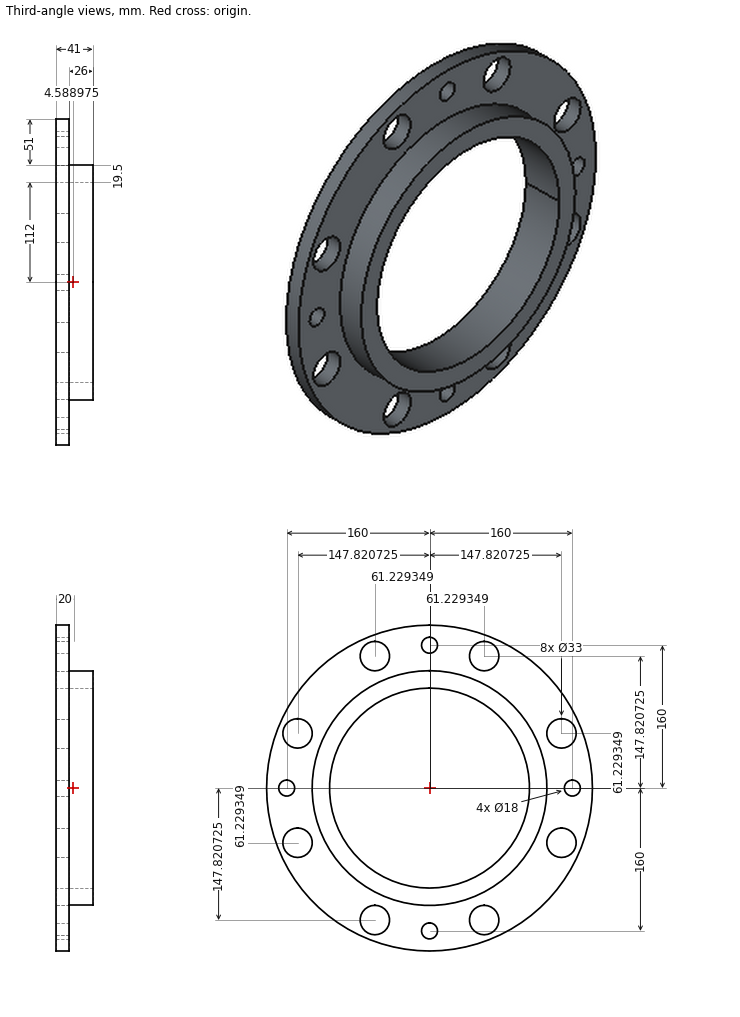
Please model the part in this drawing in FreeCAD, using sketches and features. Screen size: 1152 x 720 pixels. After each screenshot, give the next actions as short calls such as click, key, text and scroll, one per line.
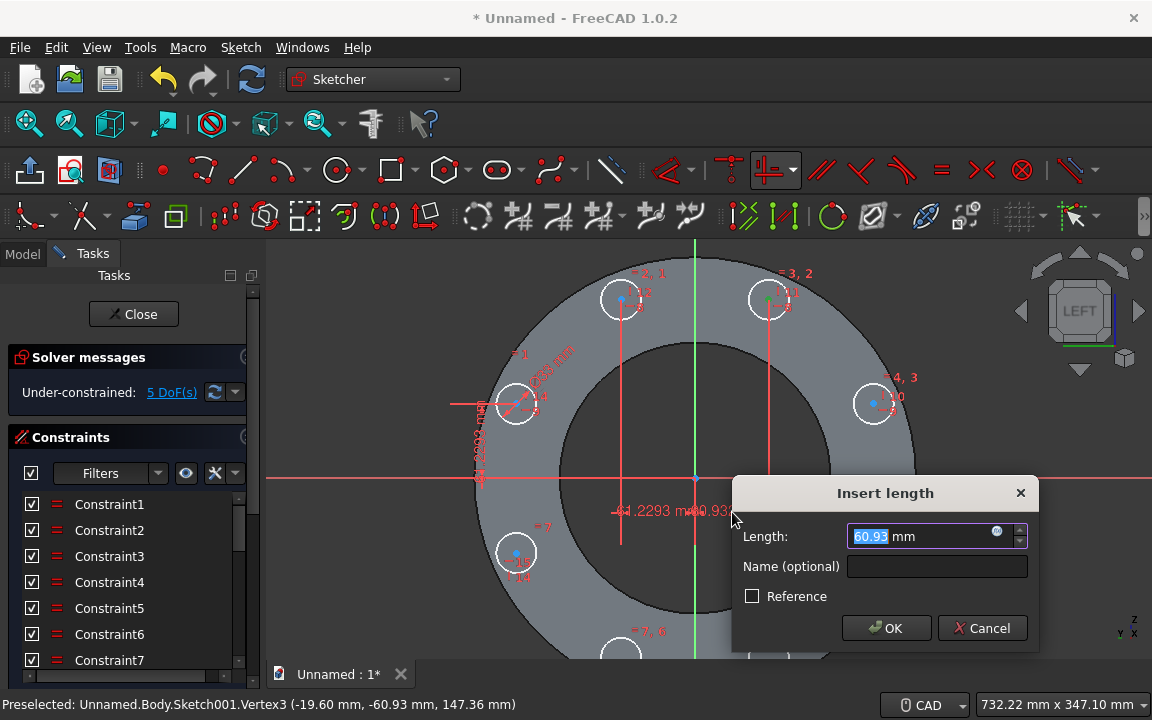
text(61.229349)
key(Return)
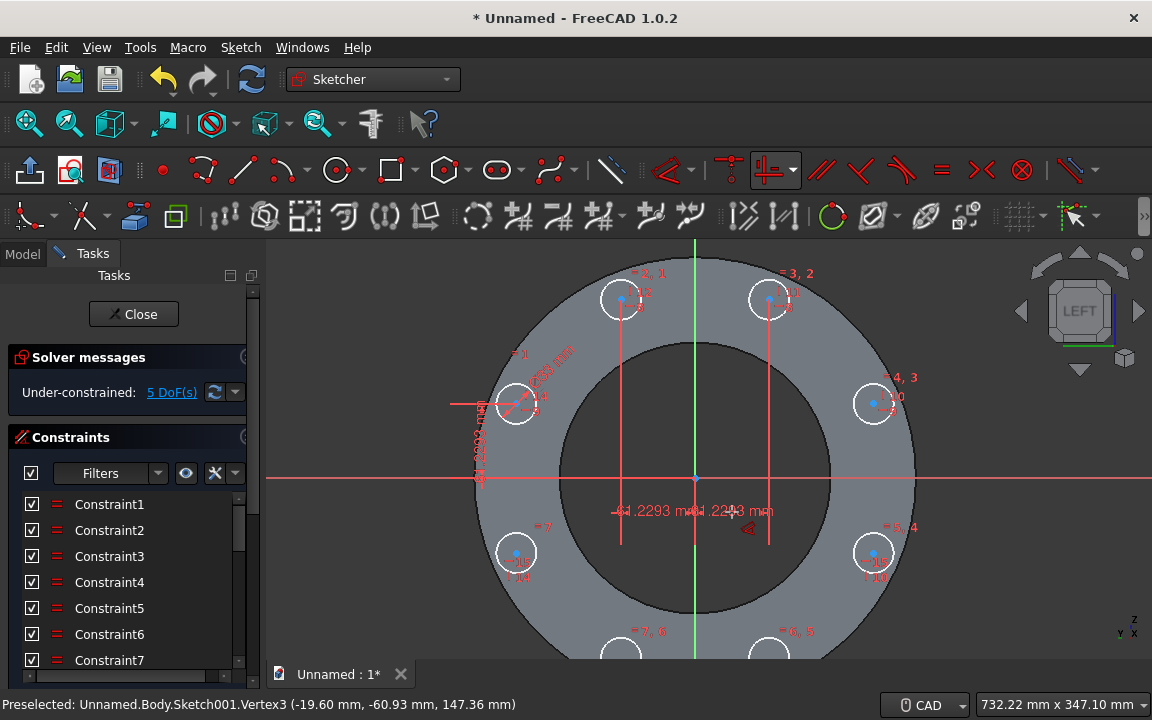
click(874, 553)
click(908, 516)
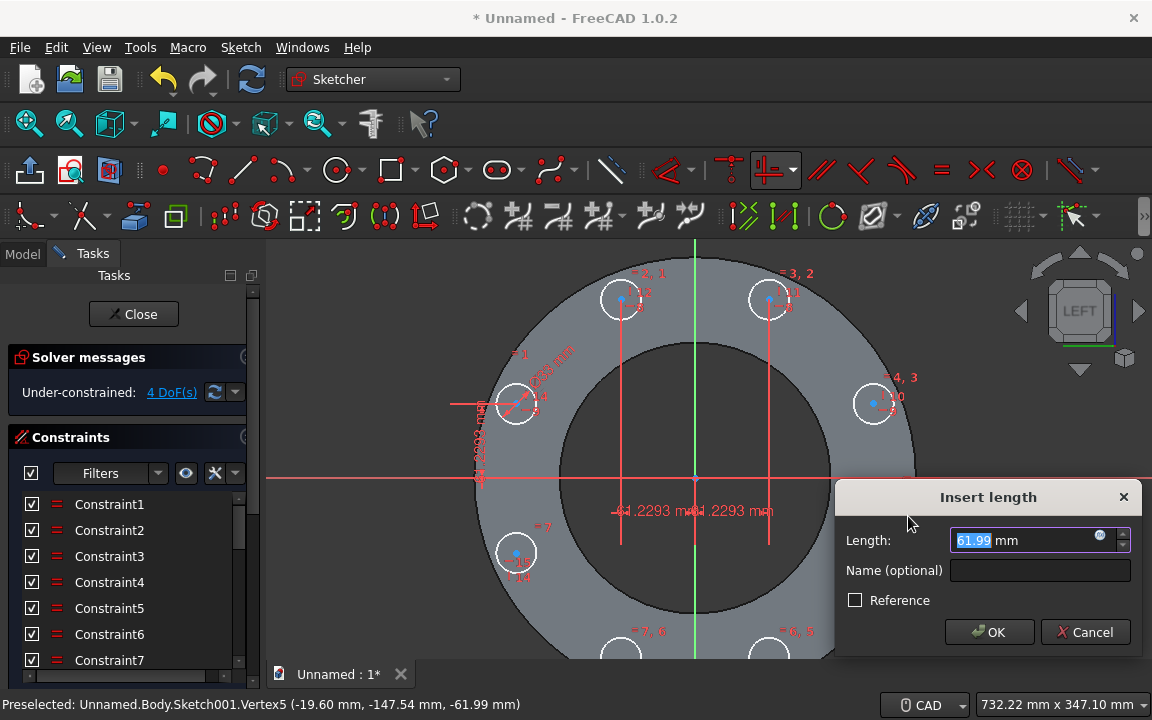
text(61.229349)
key(Return)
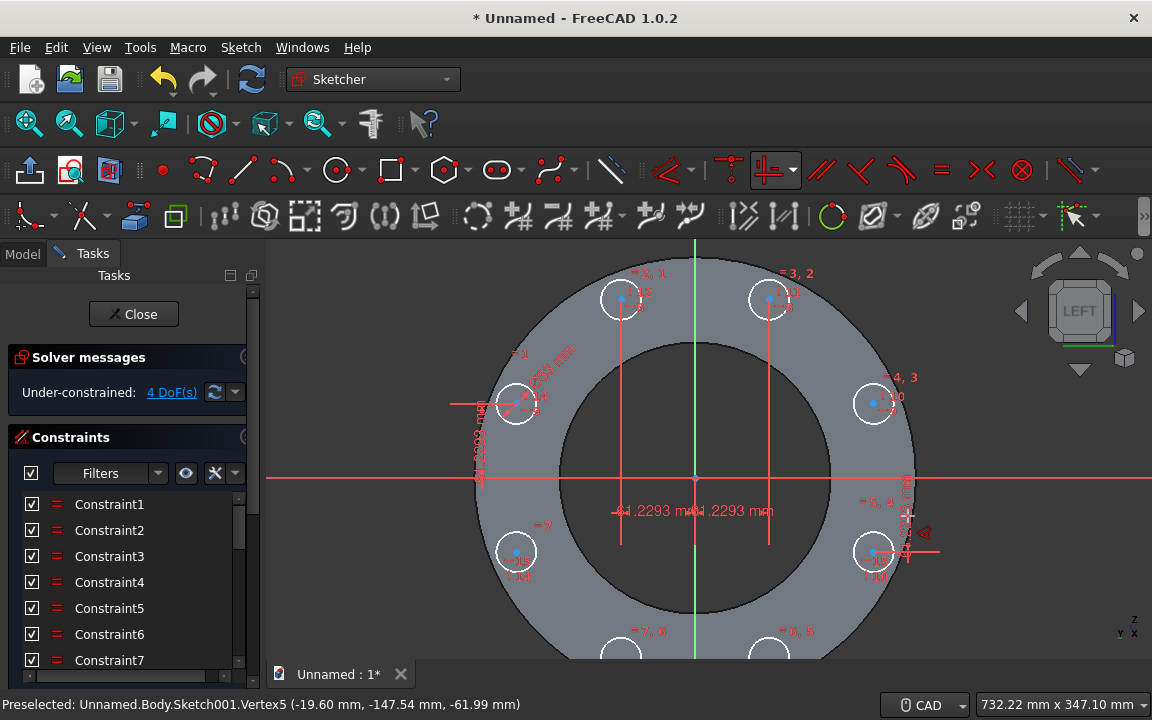
click(516, 404)
click(647, 370)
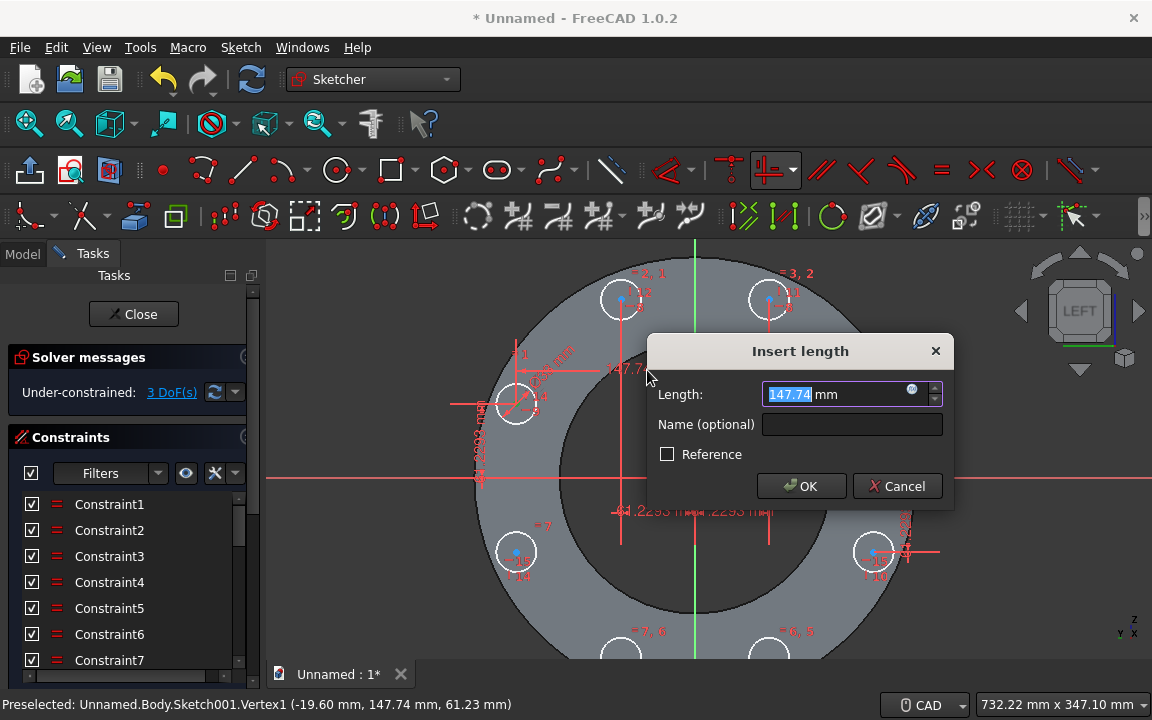
text(147.820725)
key(Return)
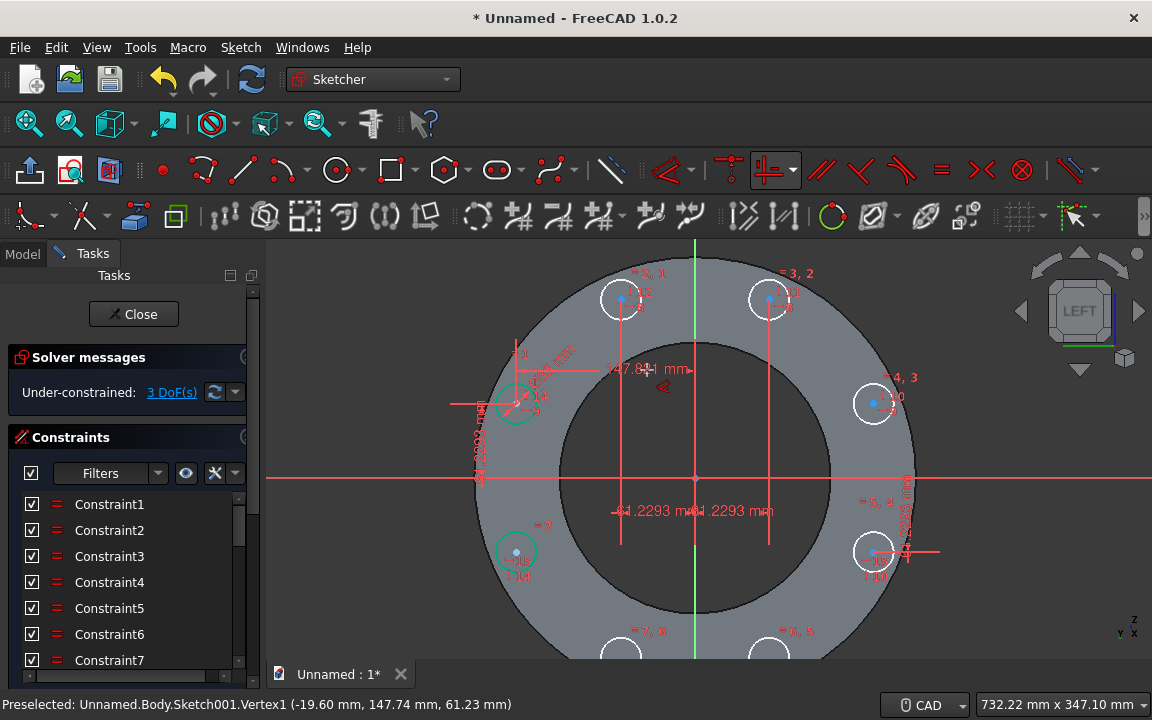
click(621, 300)
click(587, 348)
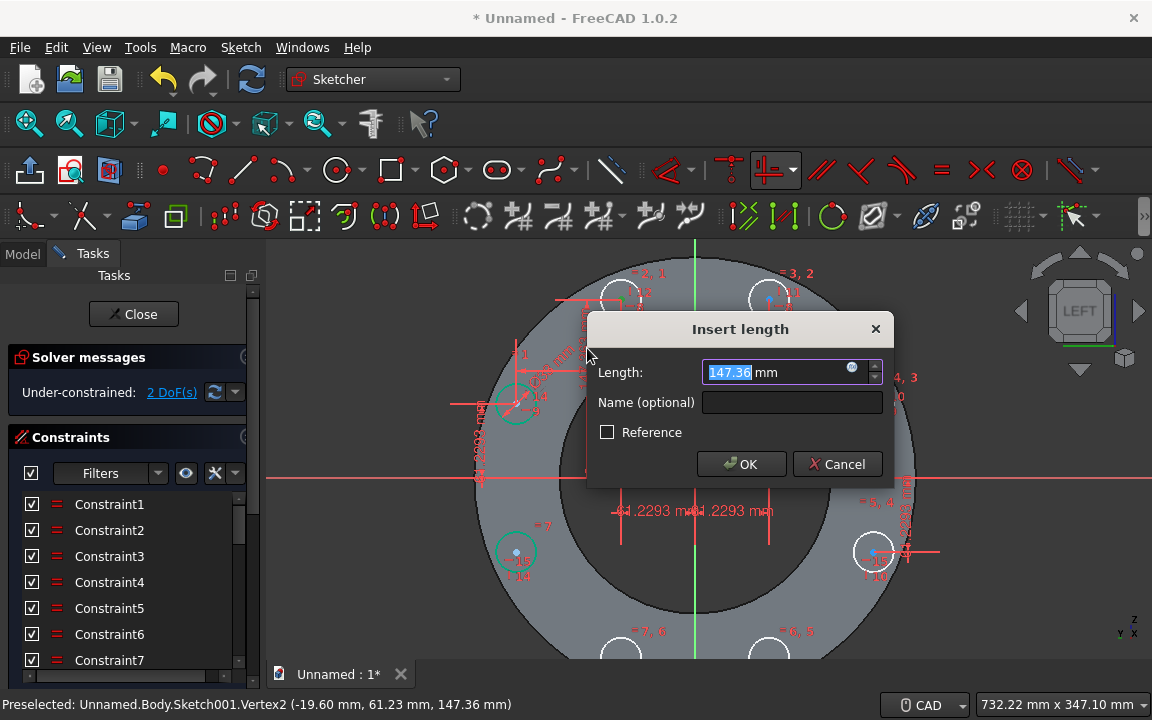
text(147.820725)
key(Return)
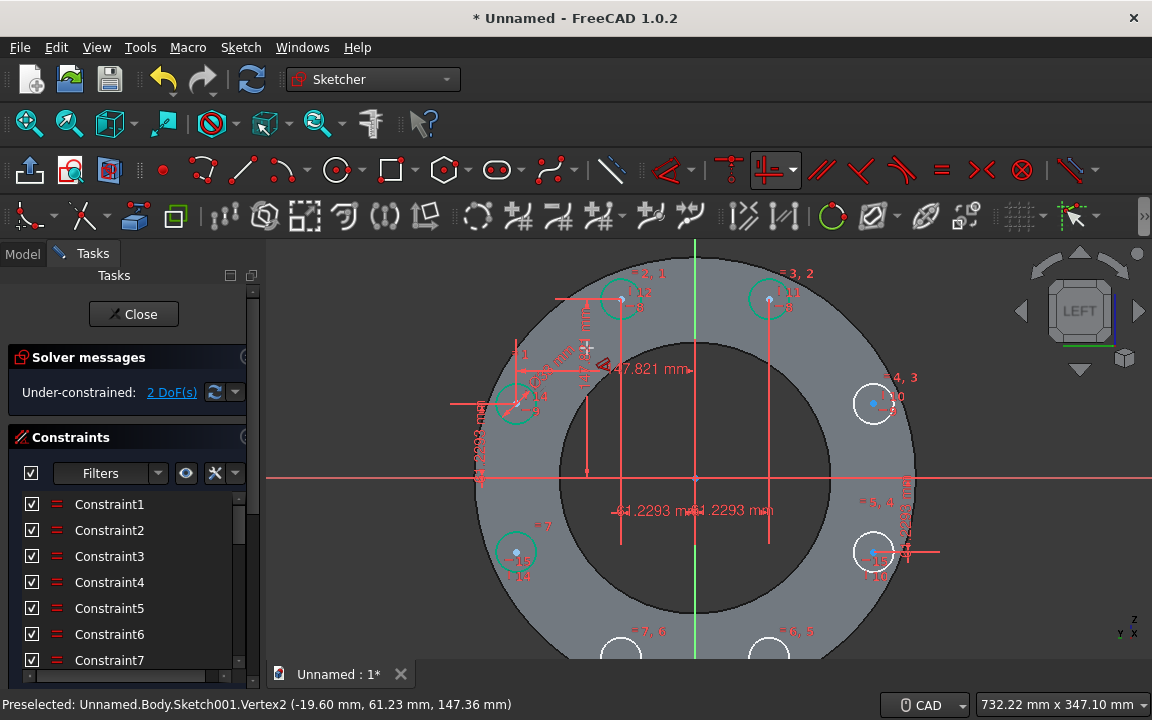
click(874, 404)
click(784, 370)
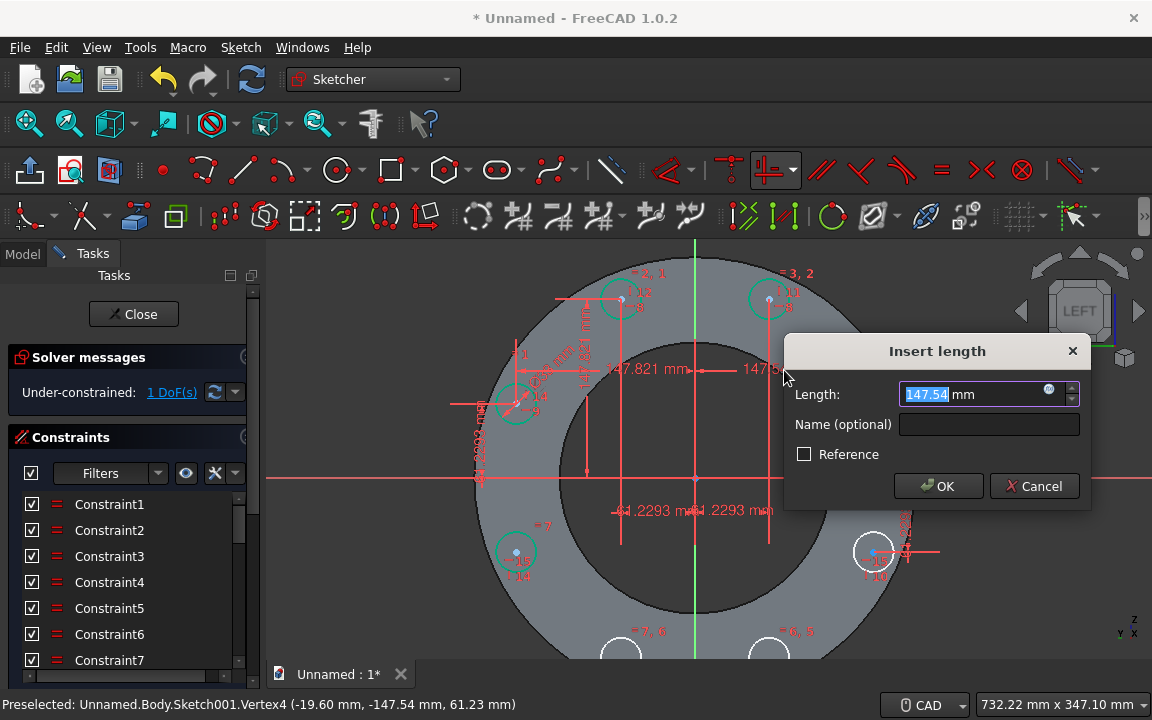
text(147.820725)
key(Return)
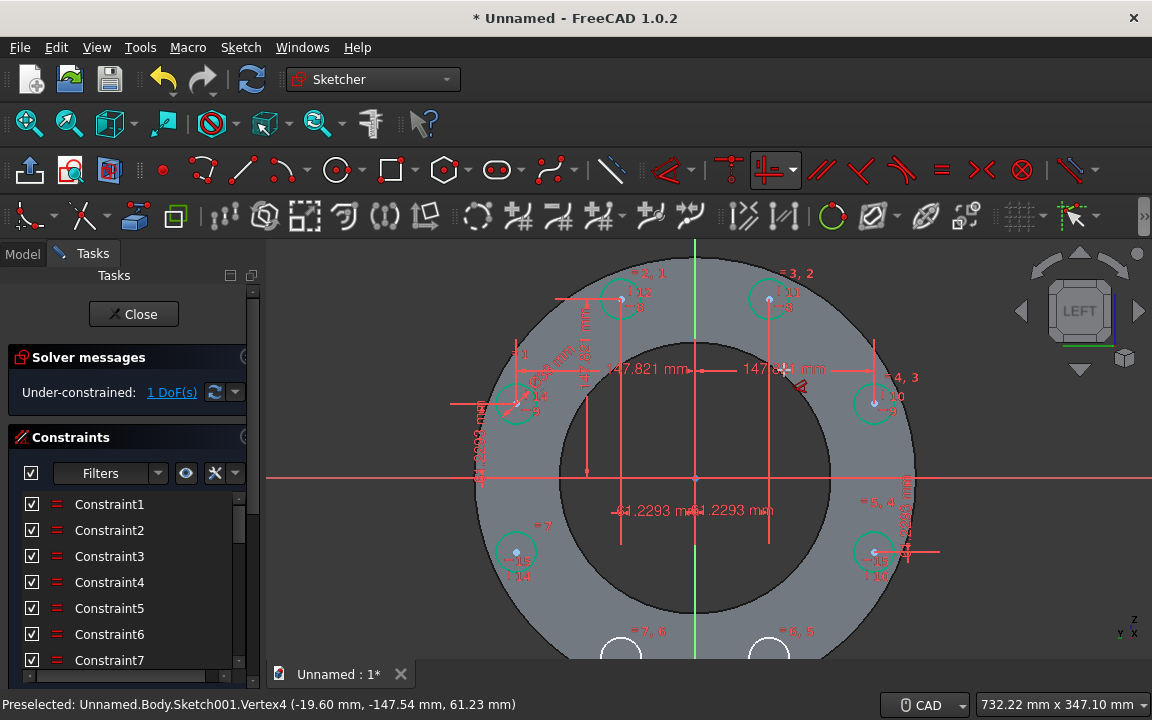
scroll(529, 390, down, 2)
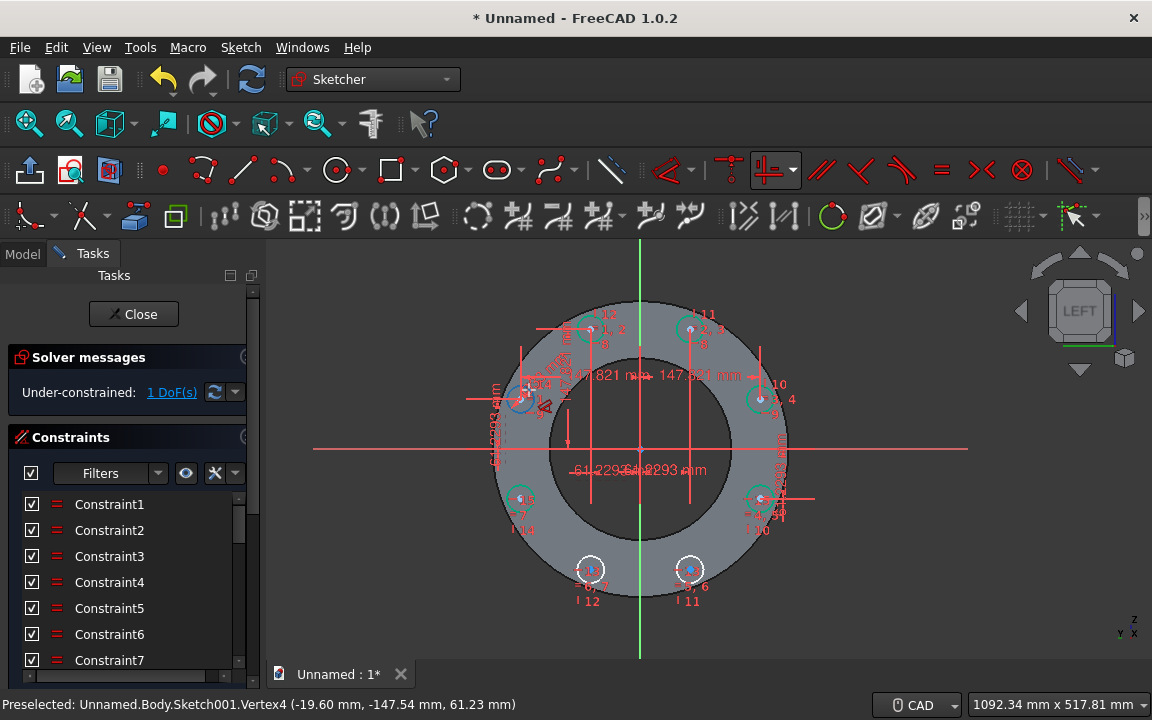
click(690, 570)
click(724, 509)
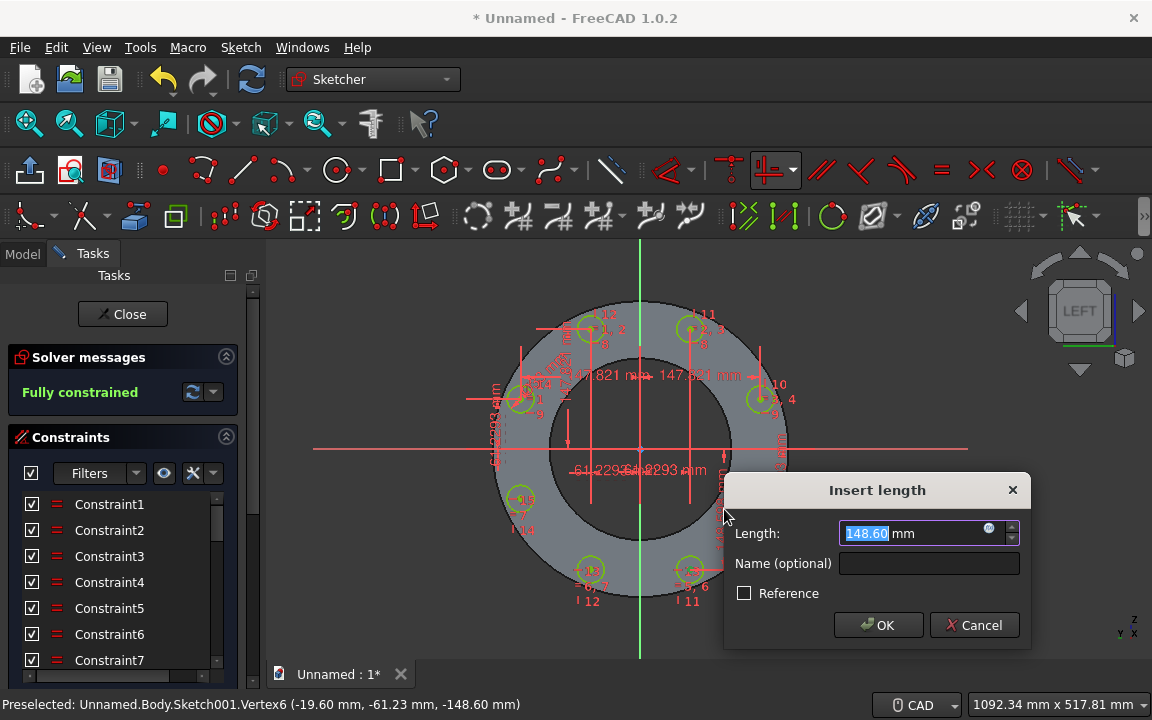
text(147.820725)
key(Return)
key(Escape)